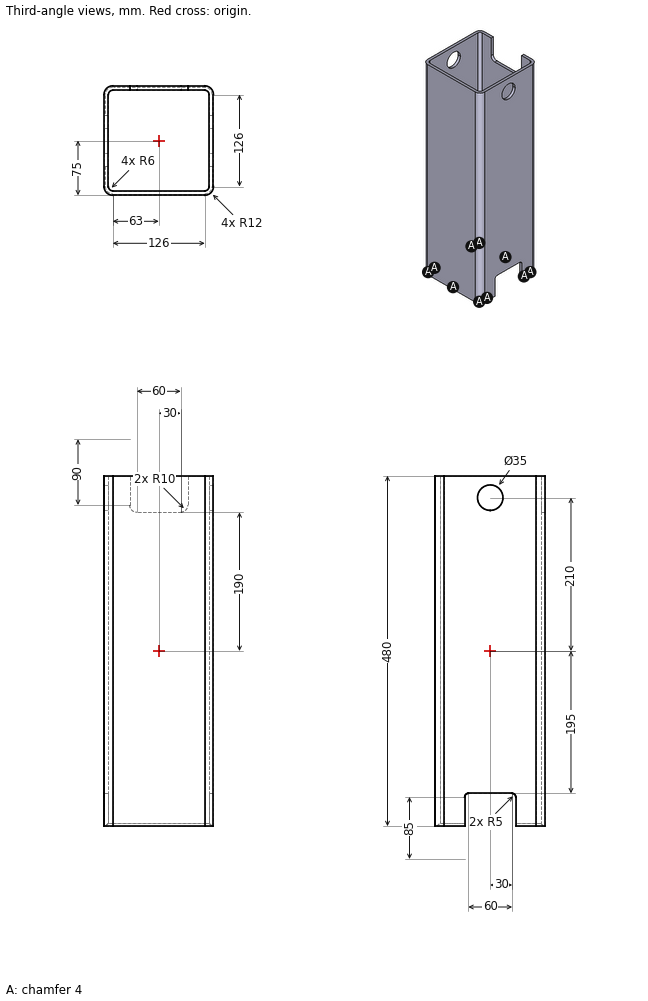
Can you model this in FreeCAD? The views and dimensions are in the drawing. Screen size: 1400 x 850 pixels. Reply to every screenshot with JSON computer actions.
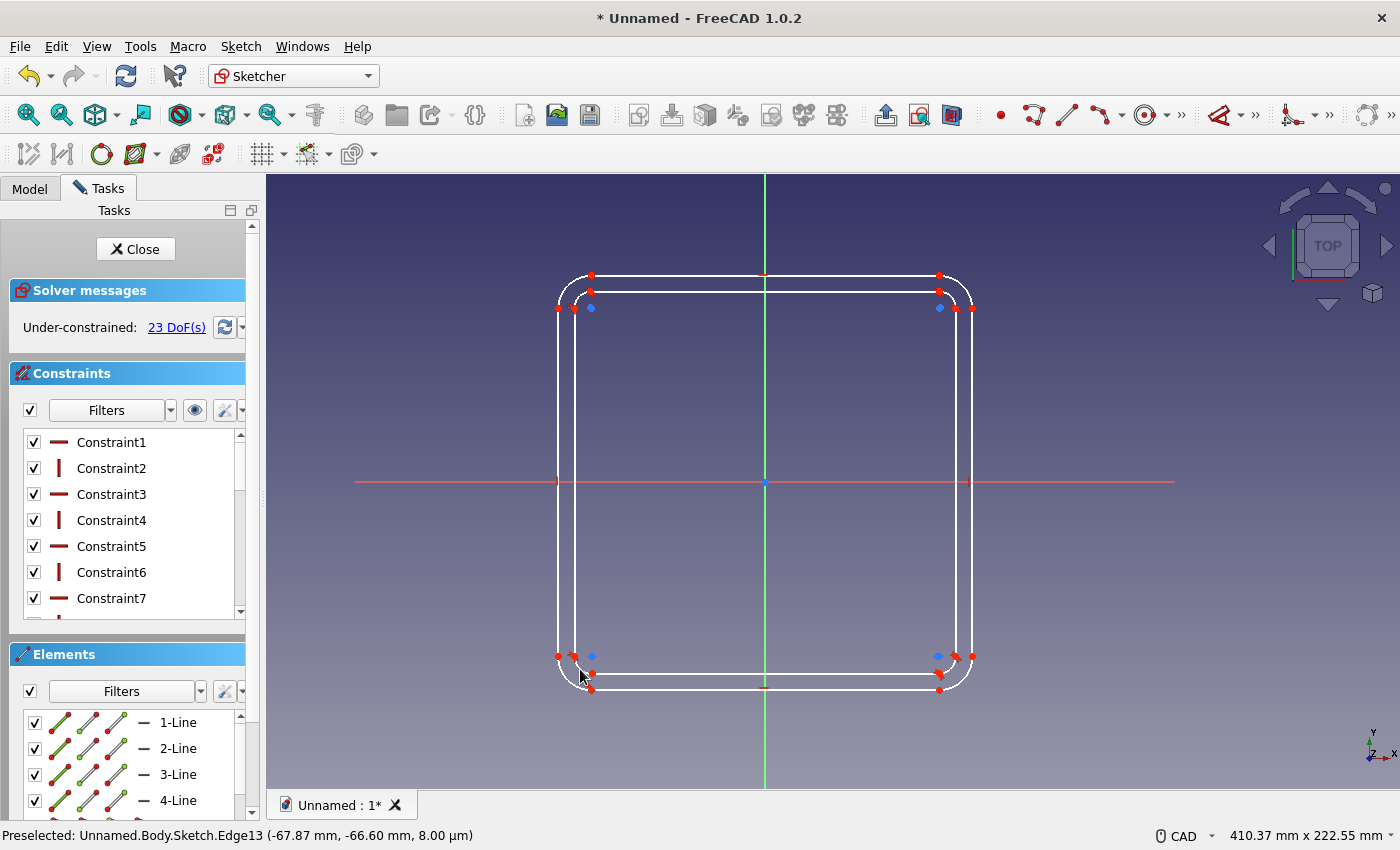
{"action": "left_click", "coordinate": [836, 674]}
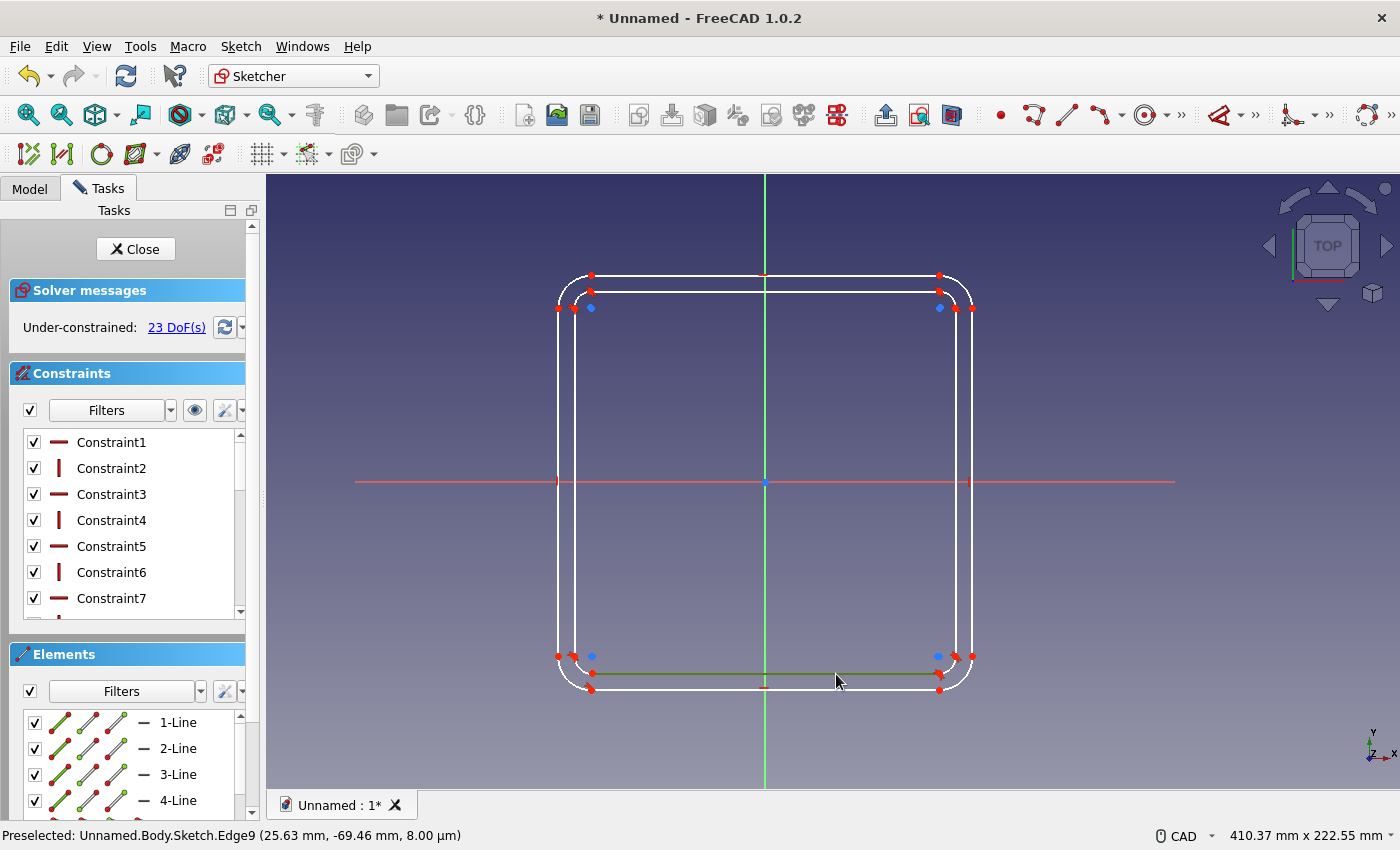
{"action": "left_click", "coordinate": [951, 668]}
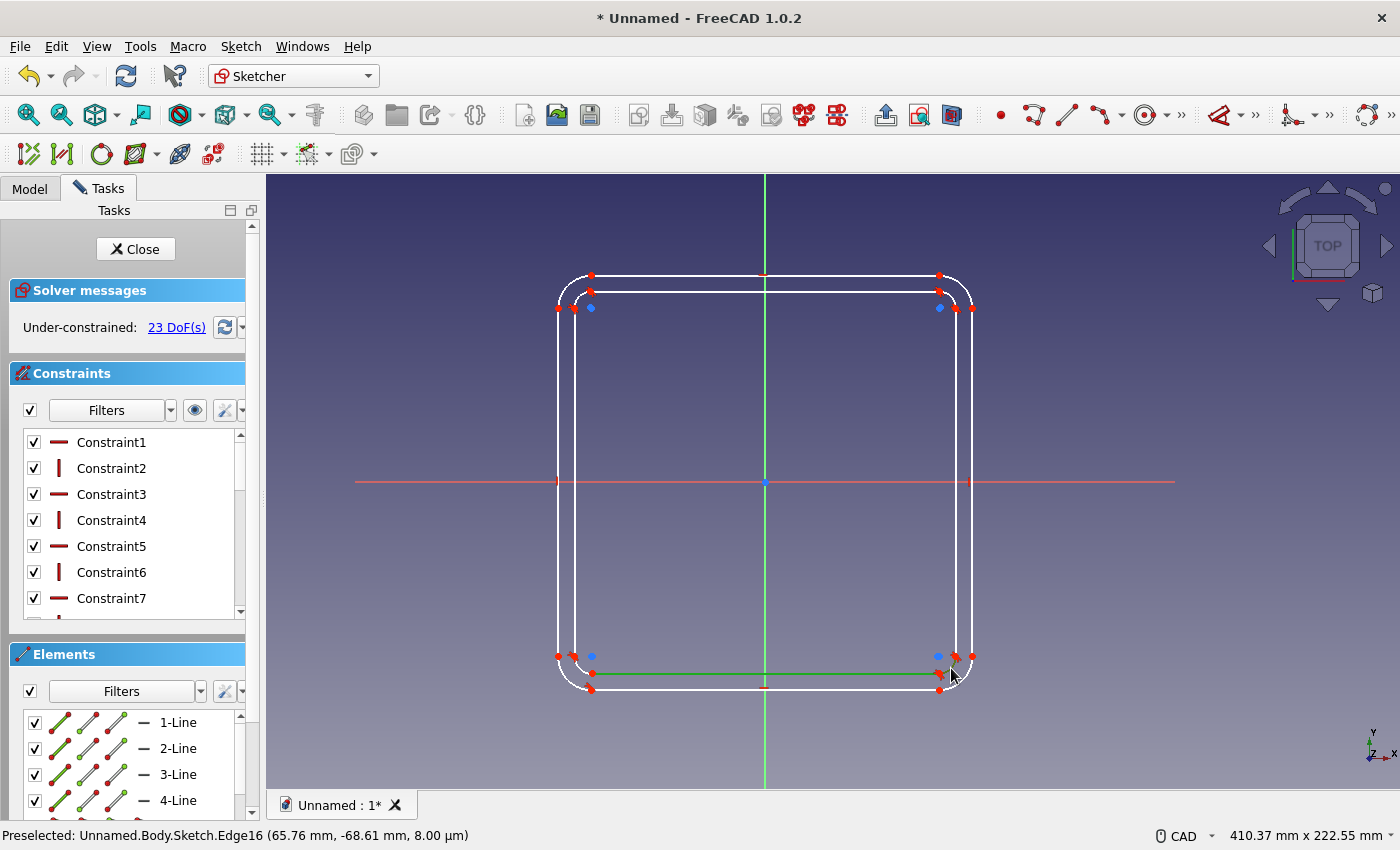
{"action": "key", "text": "t"}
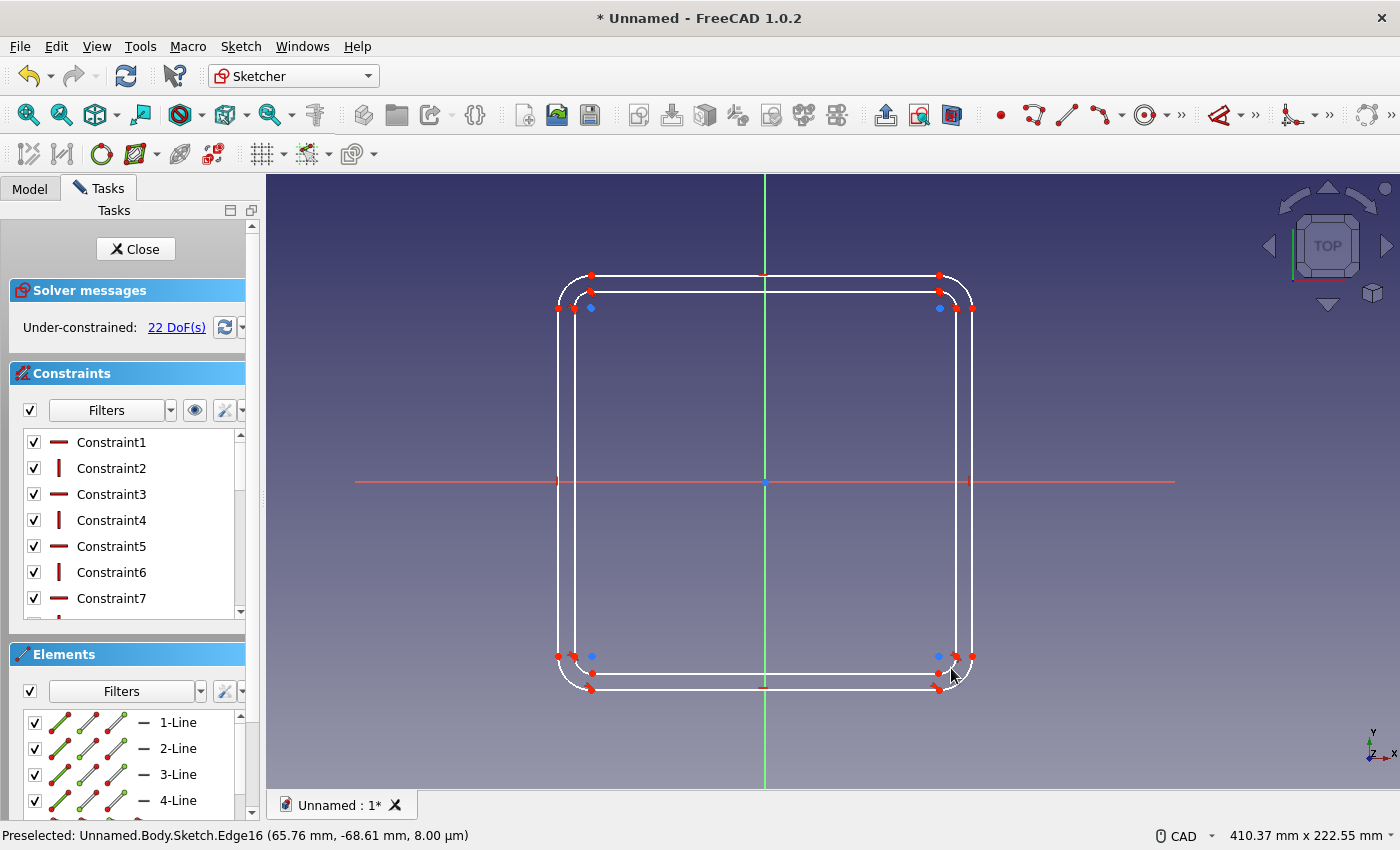
{"action": "left_click", "coordinate": [575, 553]}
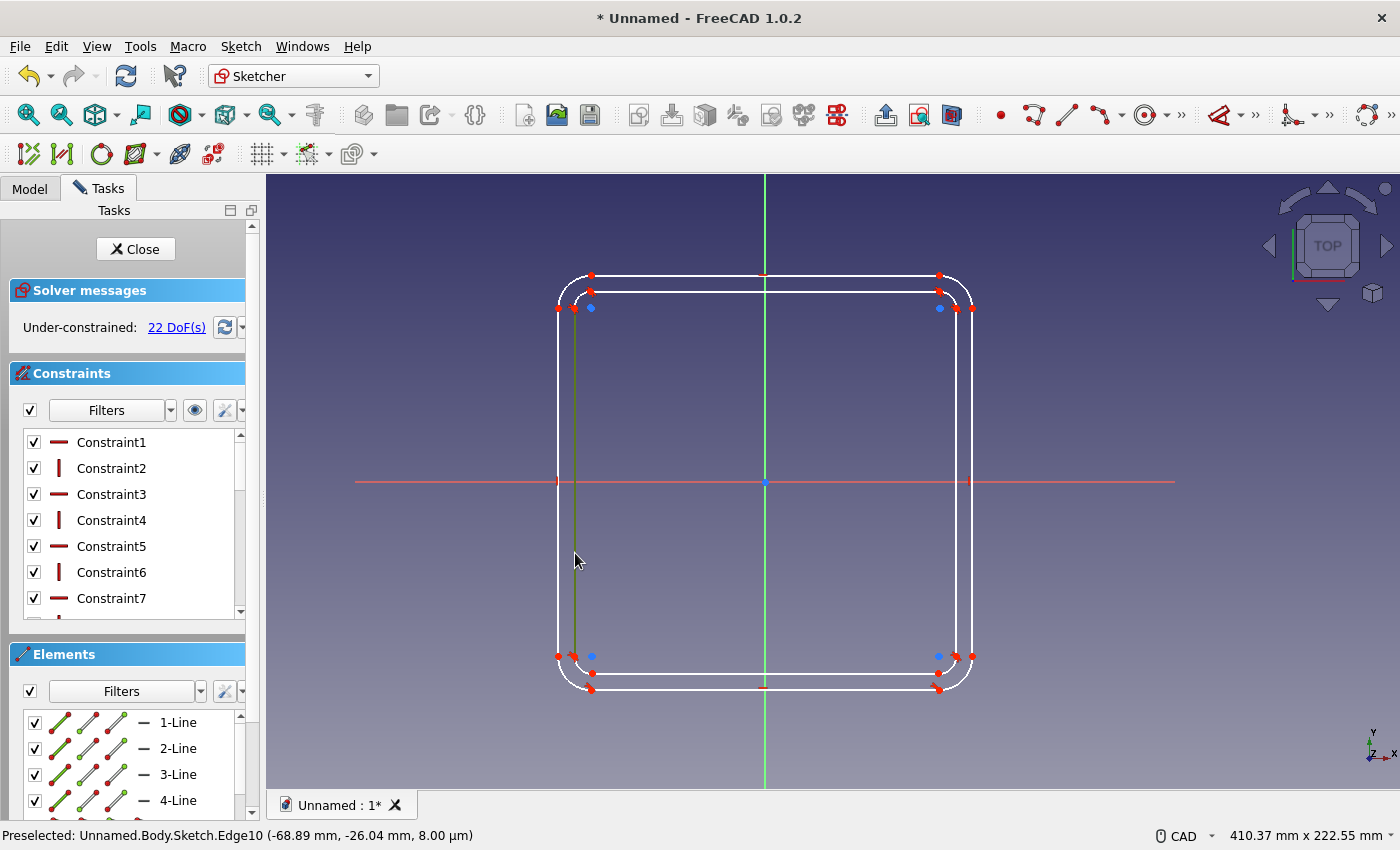
{"action": "left_click", "coordinate": [580, 669]}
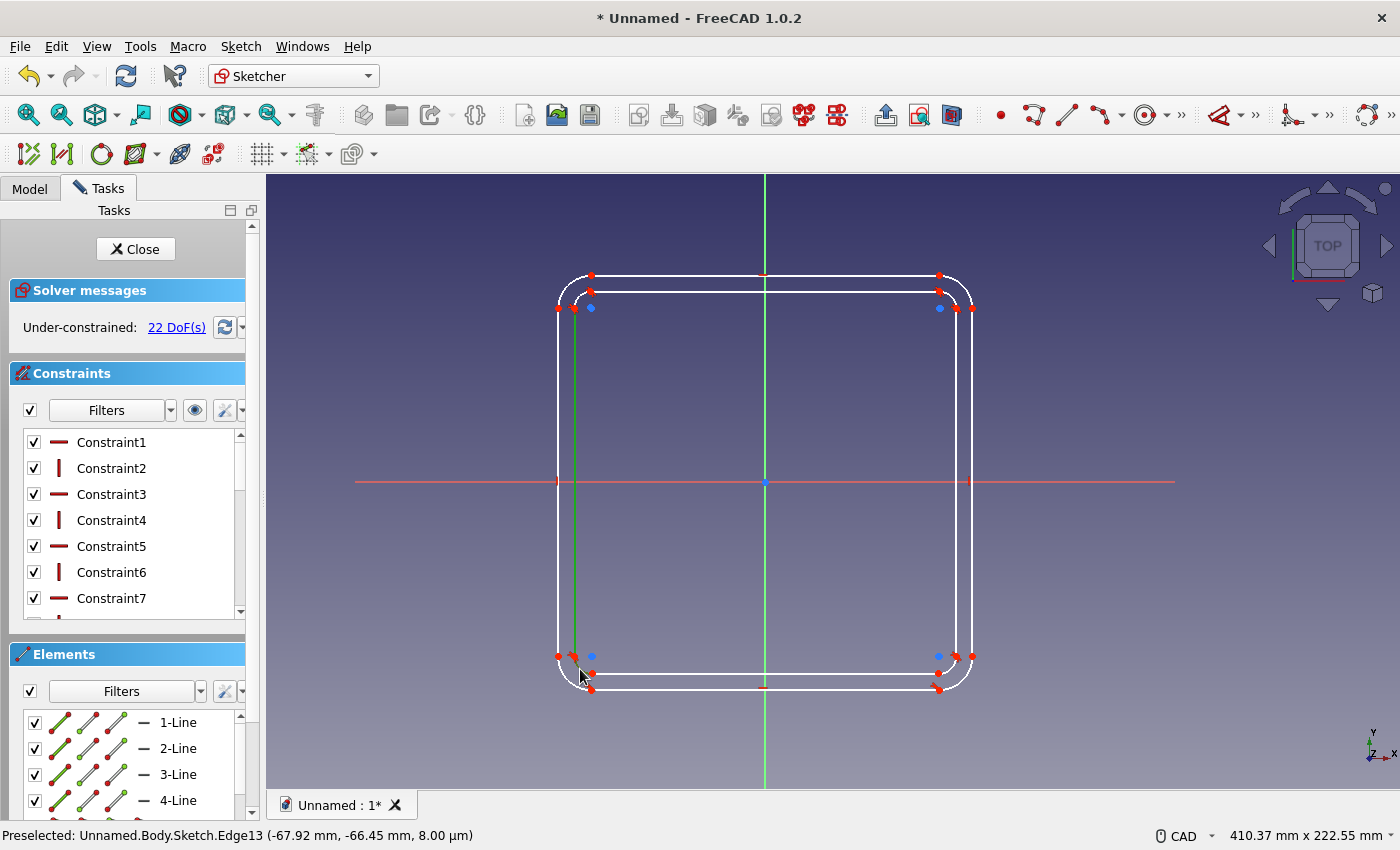
{"action": "key", "text": "t"}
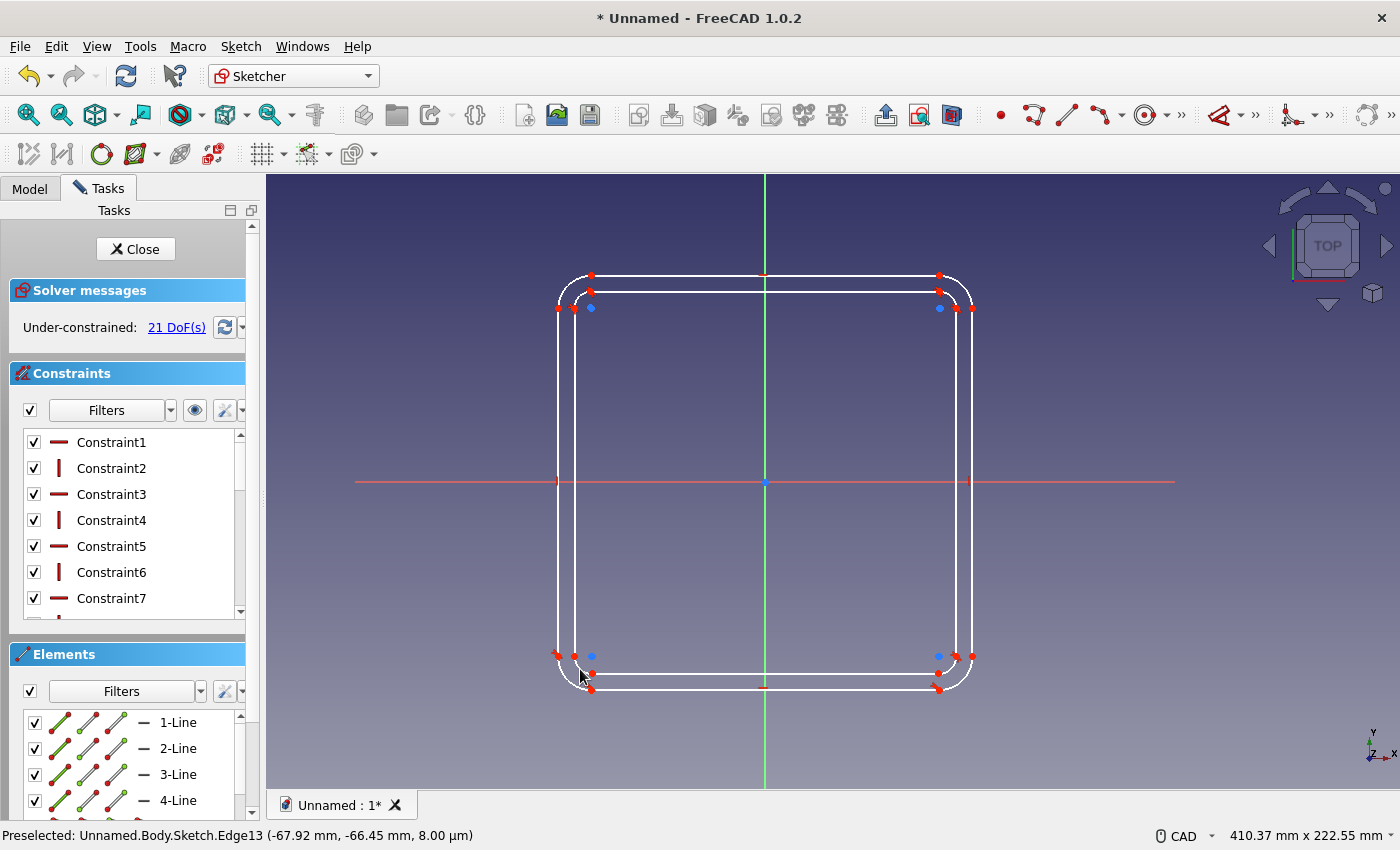
{"action": "left_click", "coordinate": [575, 552]}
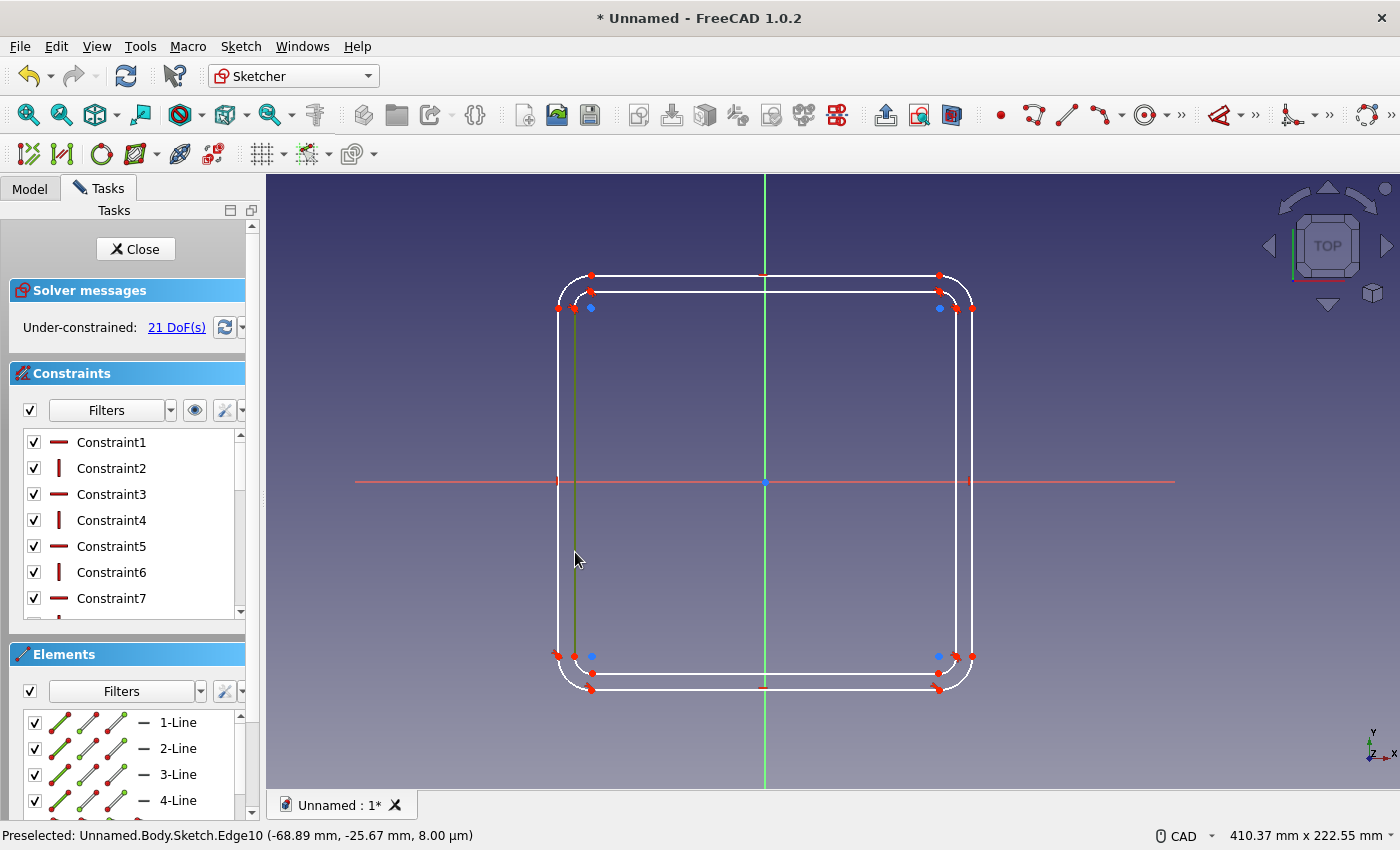
{"action": "left_click", "coordinate": [579, 297]}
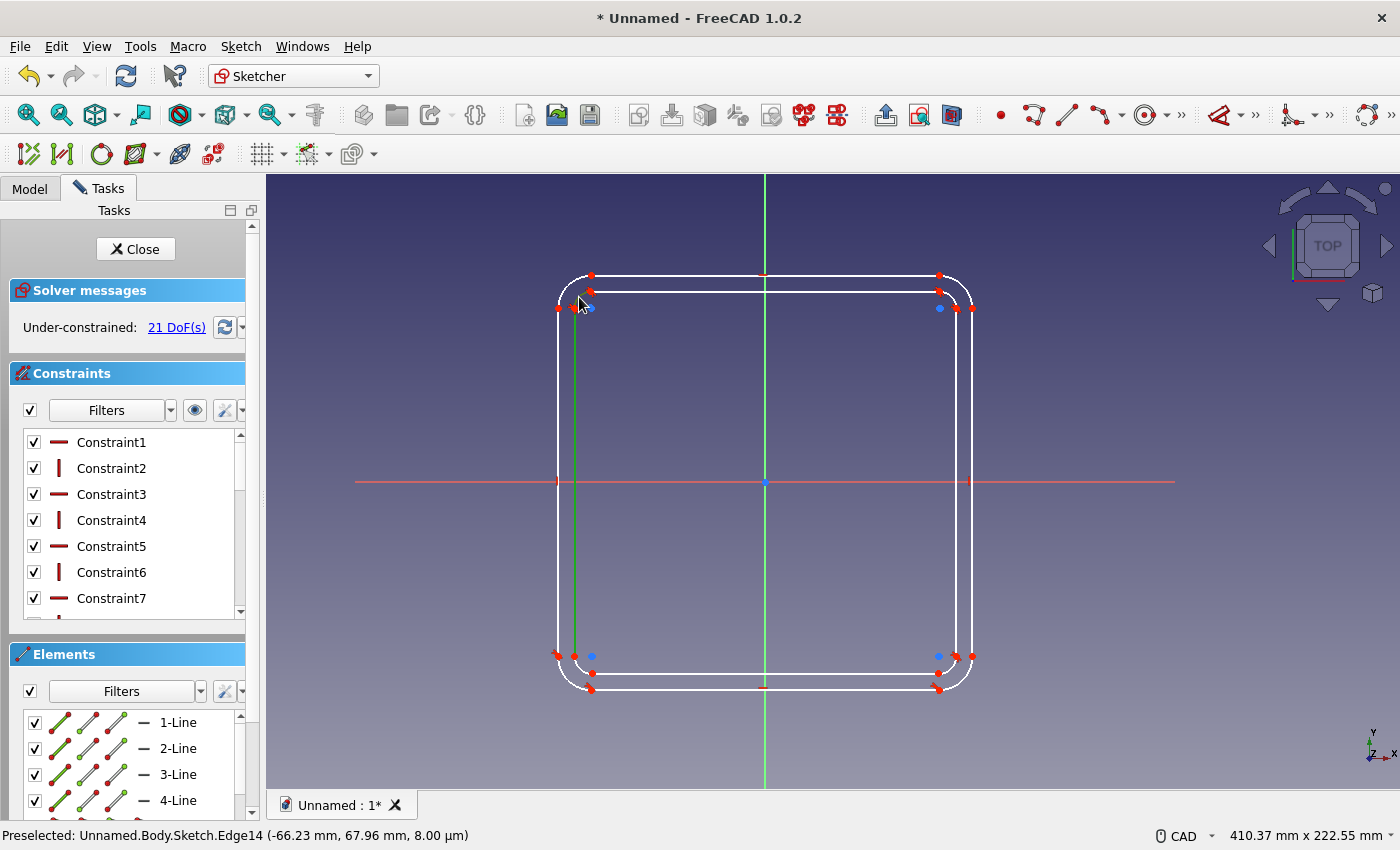
{"action": "key", "text": "t"}